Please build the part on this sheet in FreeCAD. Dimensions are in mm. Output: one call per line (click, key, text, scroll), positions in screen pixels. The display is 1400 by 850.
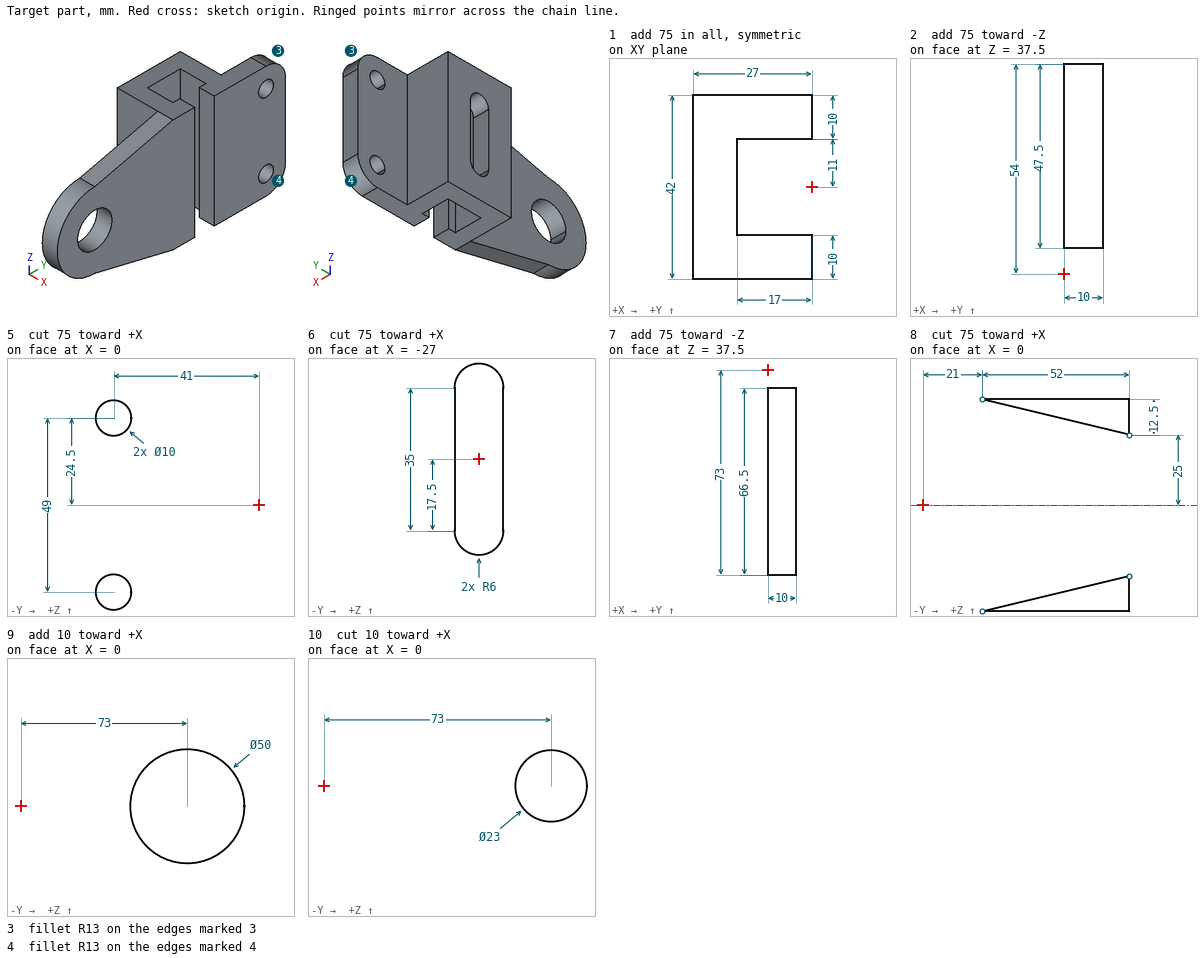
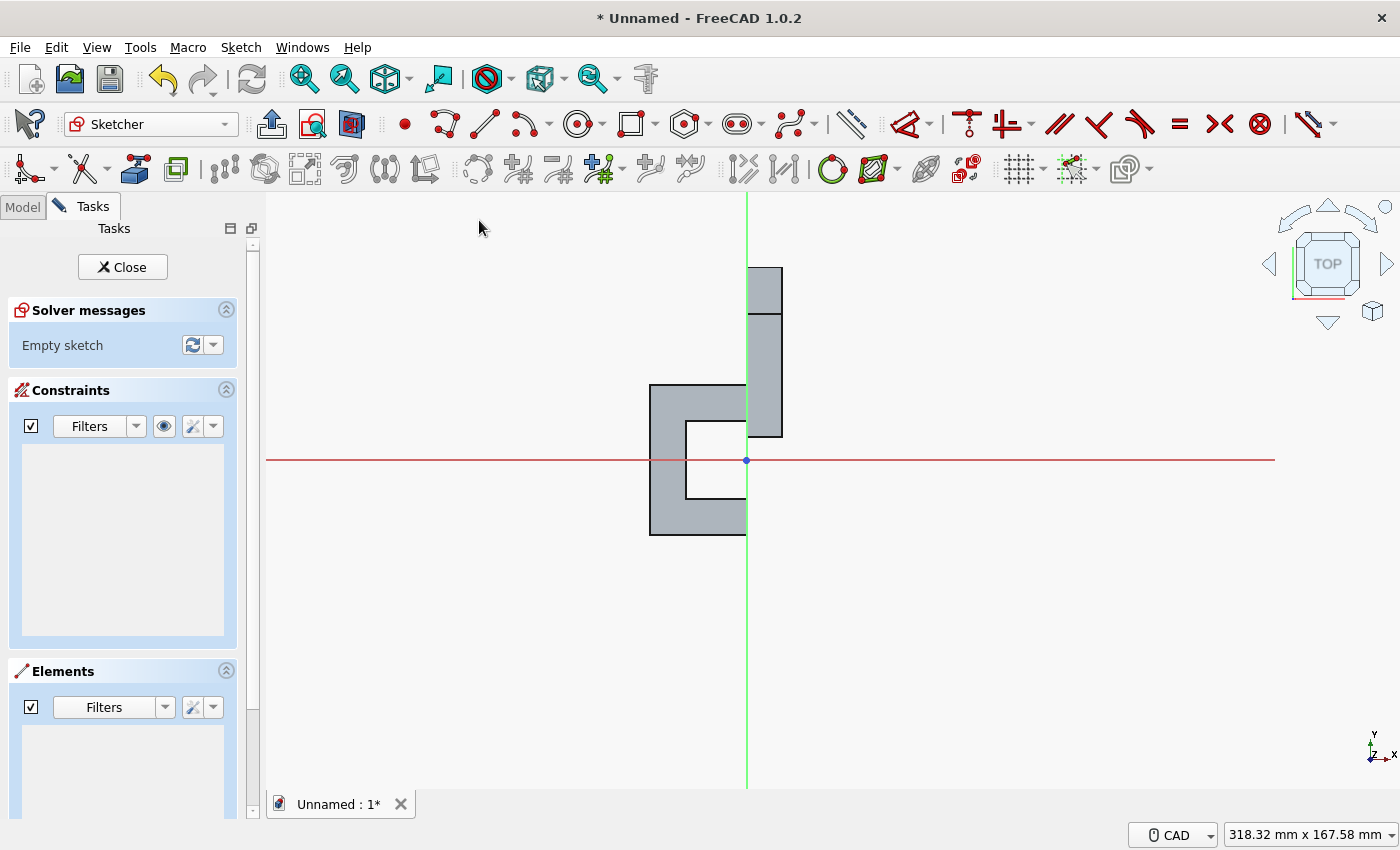
scroll(764, 761, up, 2)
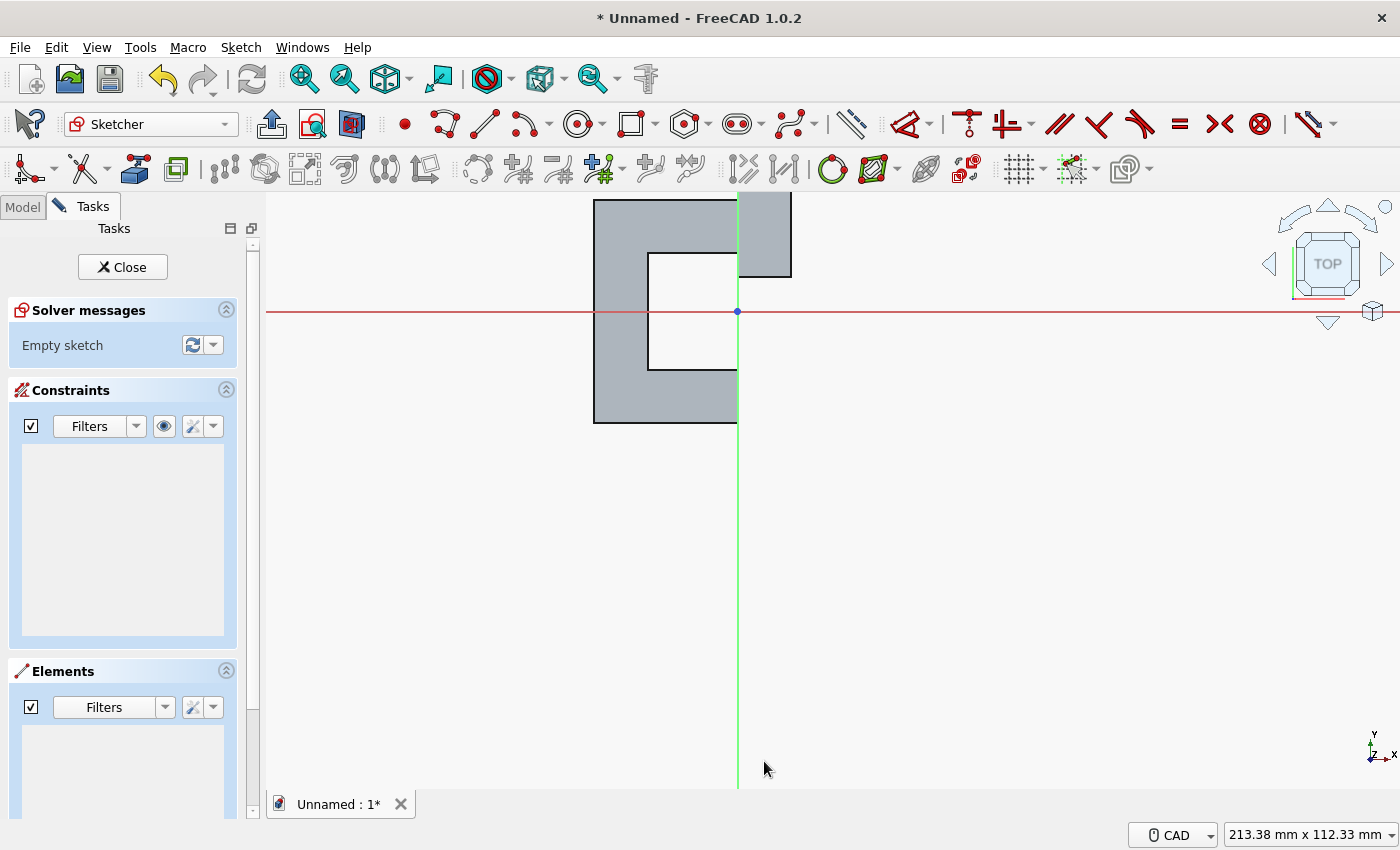
key(g)
key(r)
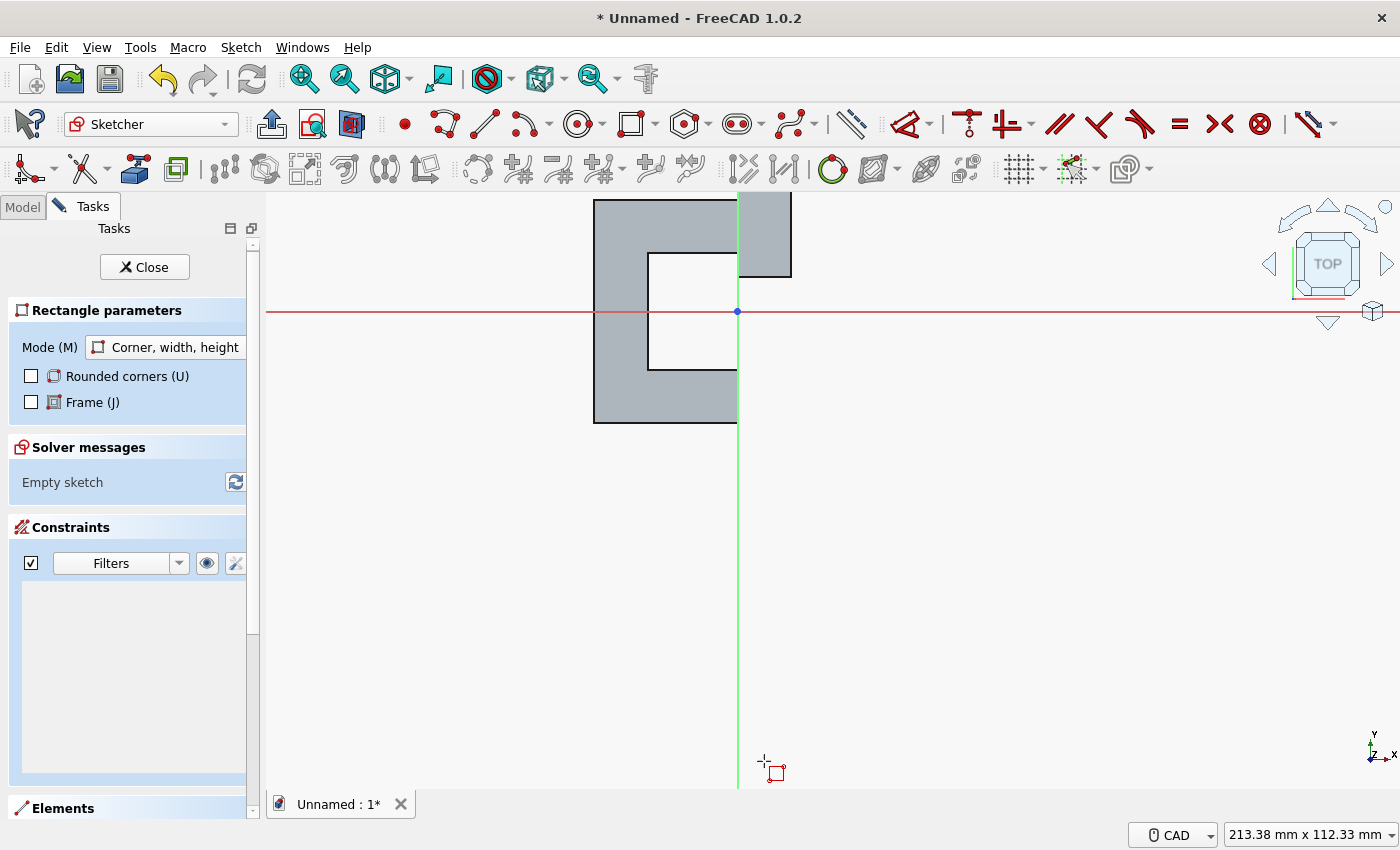
click(738, 346)
click(791, 700)
key(Escape)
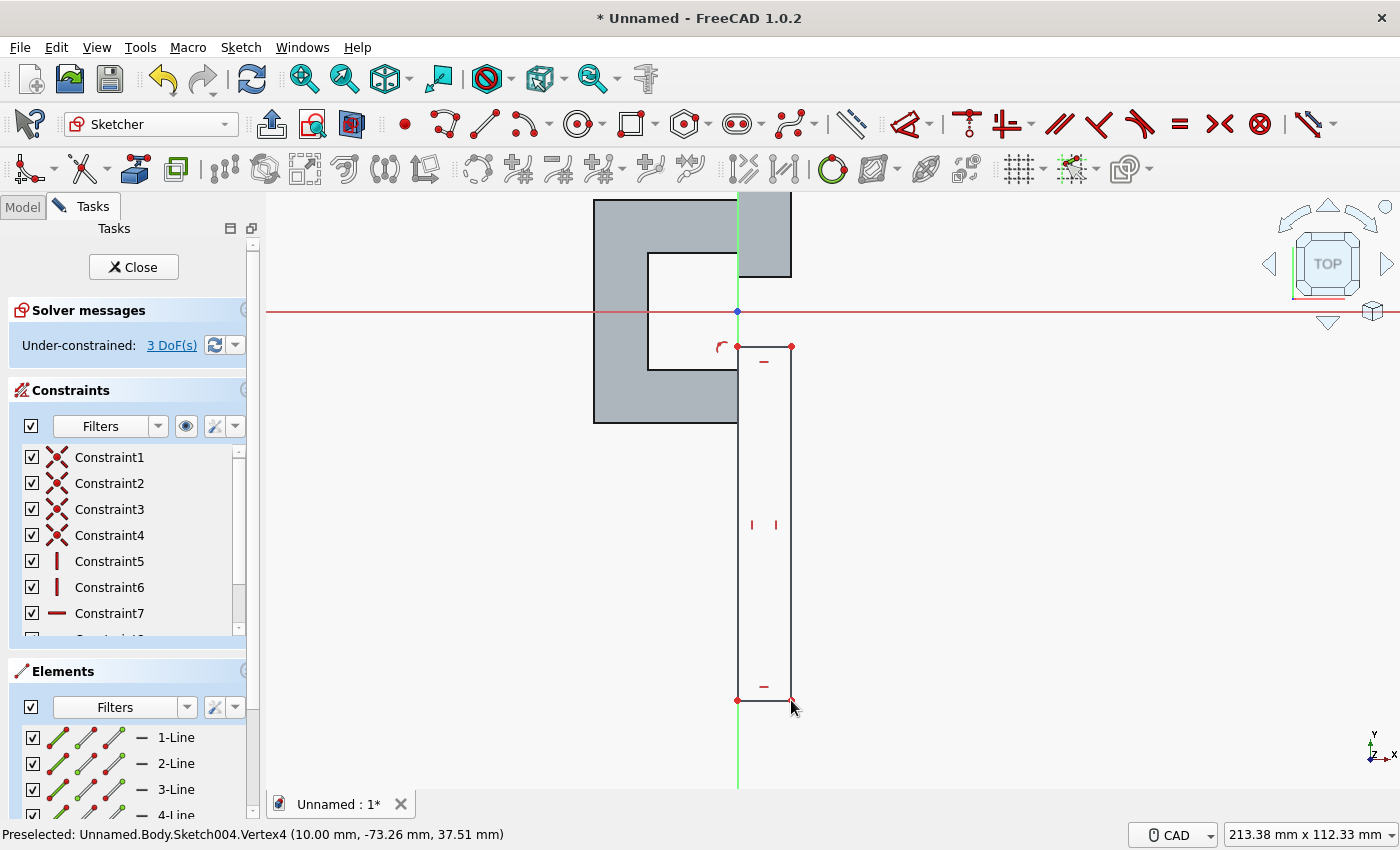
key(d)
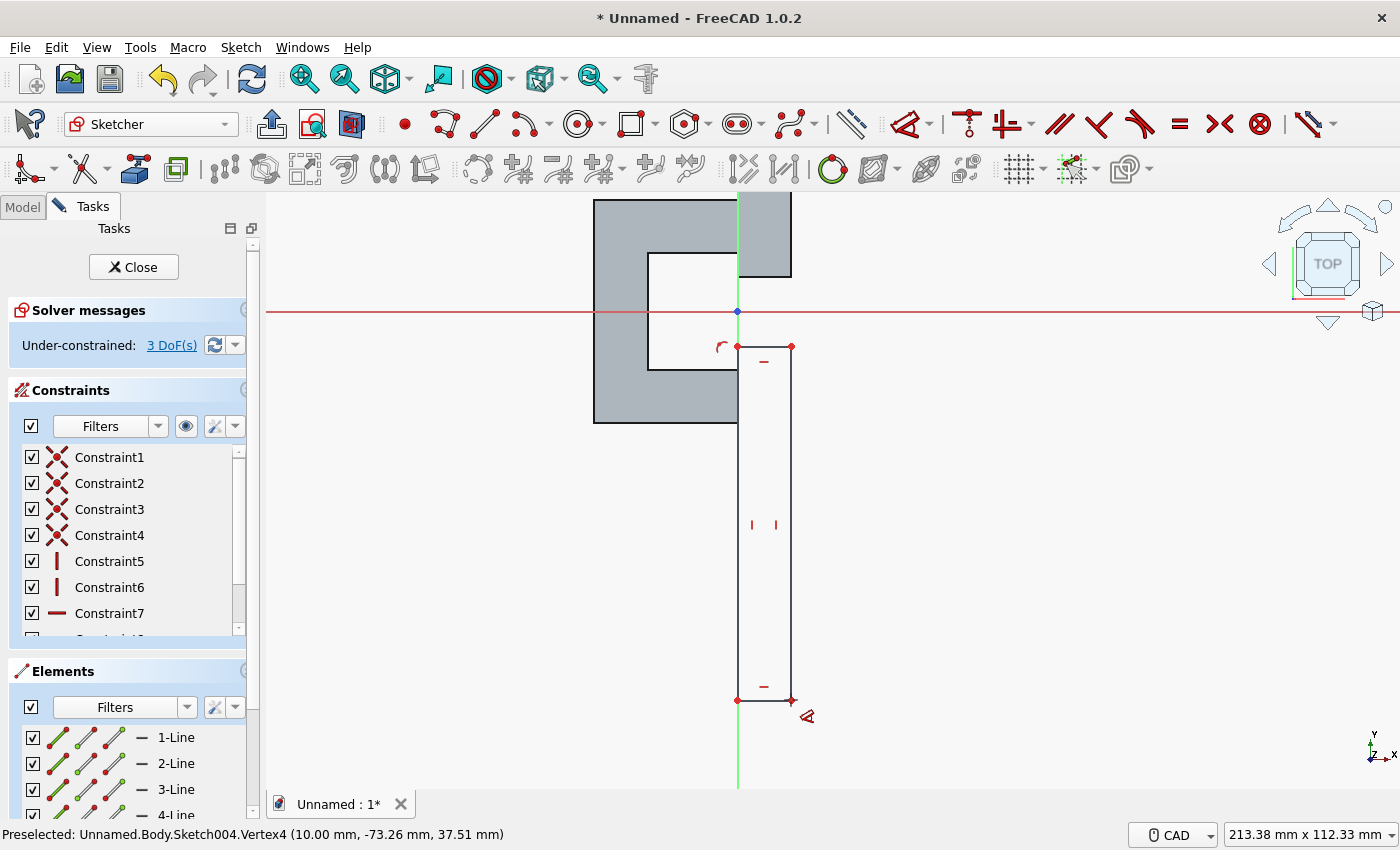
click(754, 701)
click(764, 735)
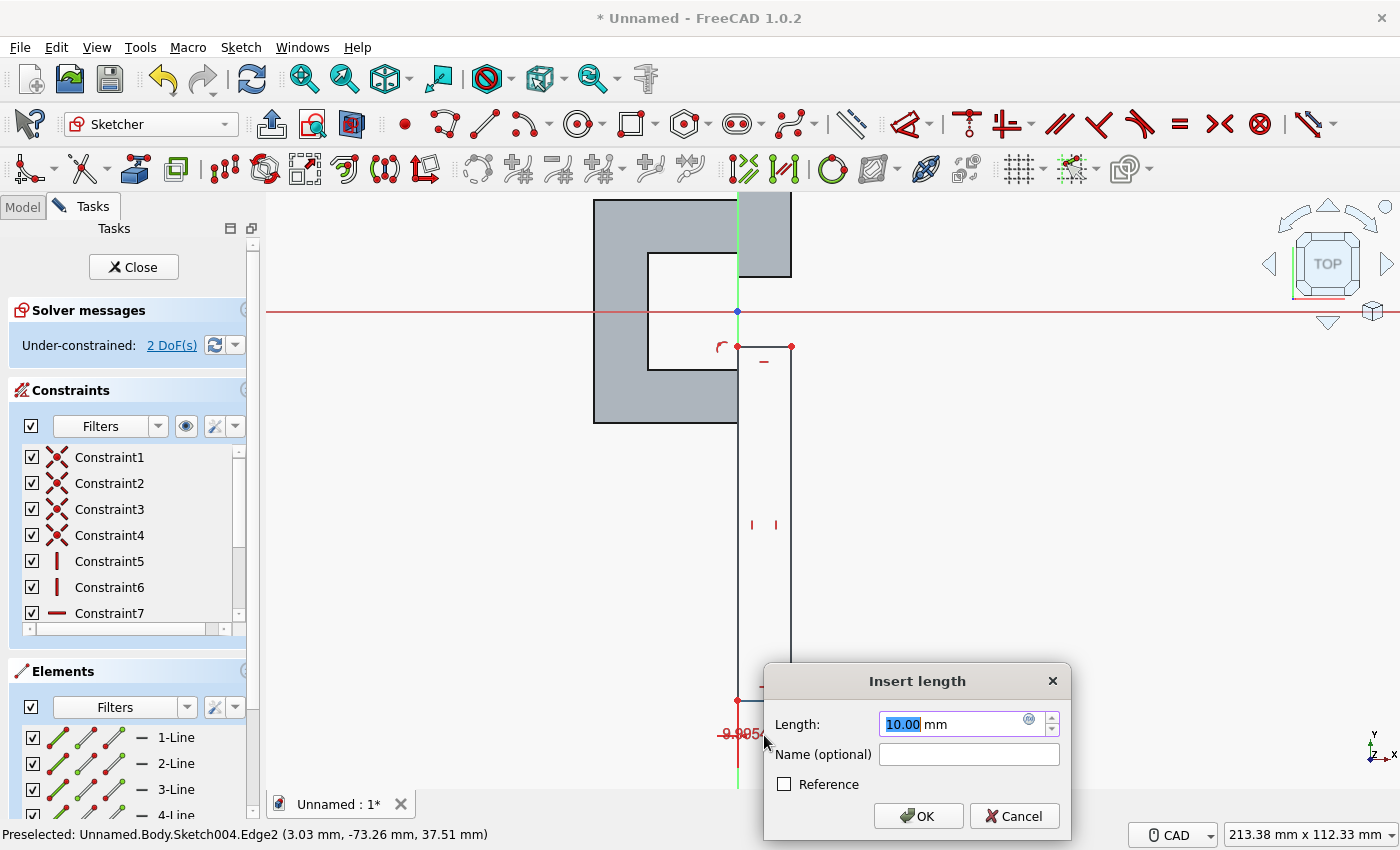
text(10)
key(Return)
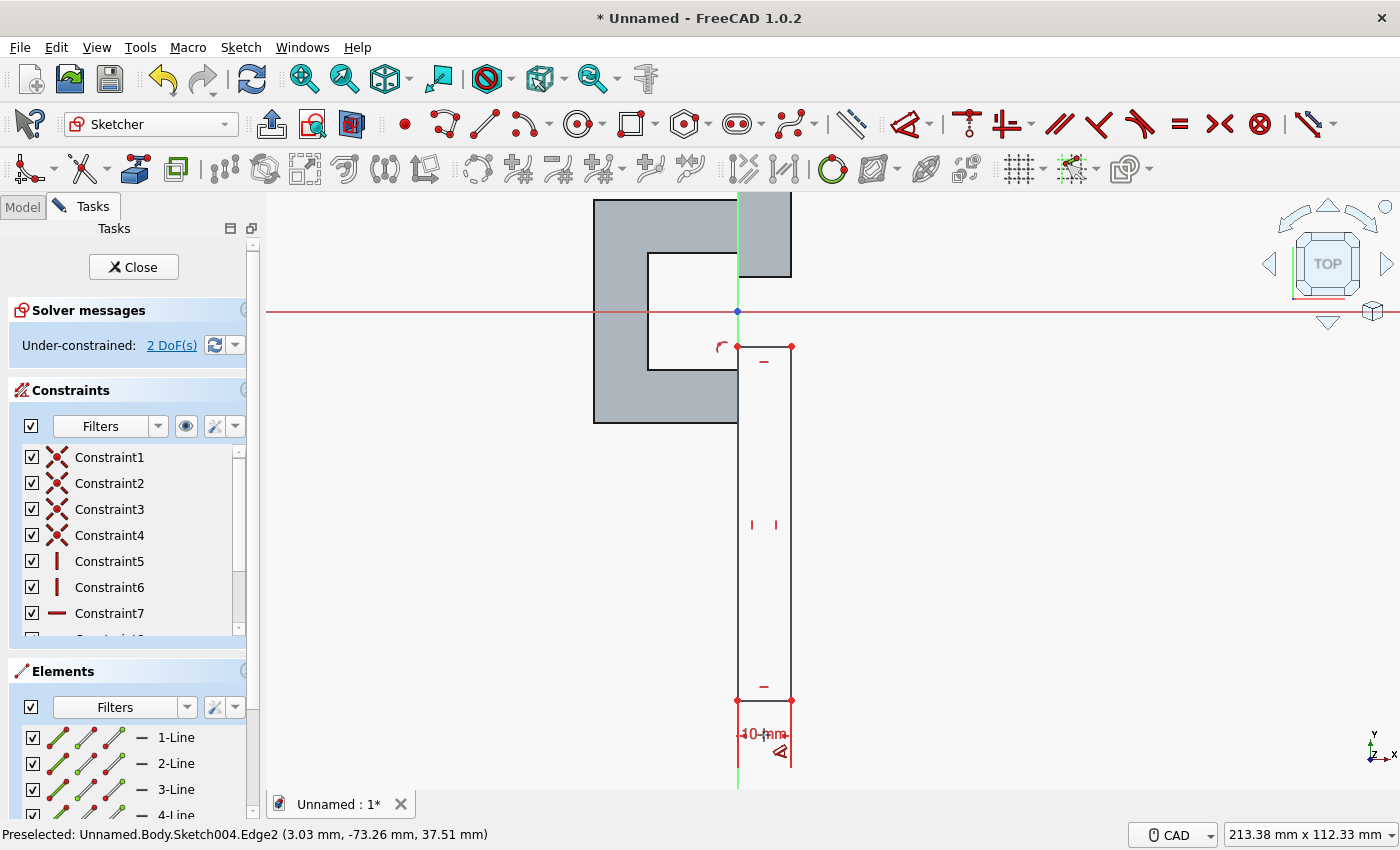
click(738, 701)
click(704, 506)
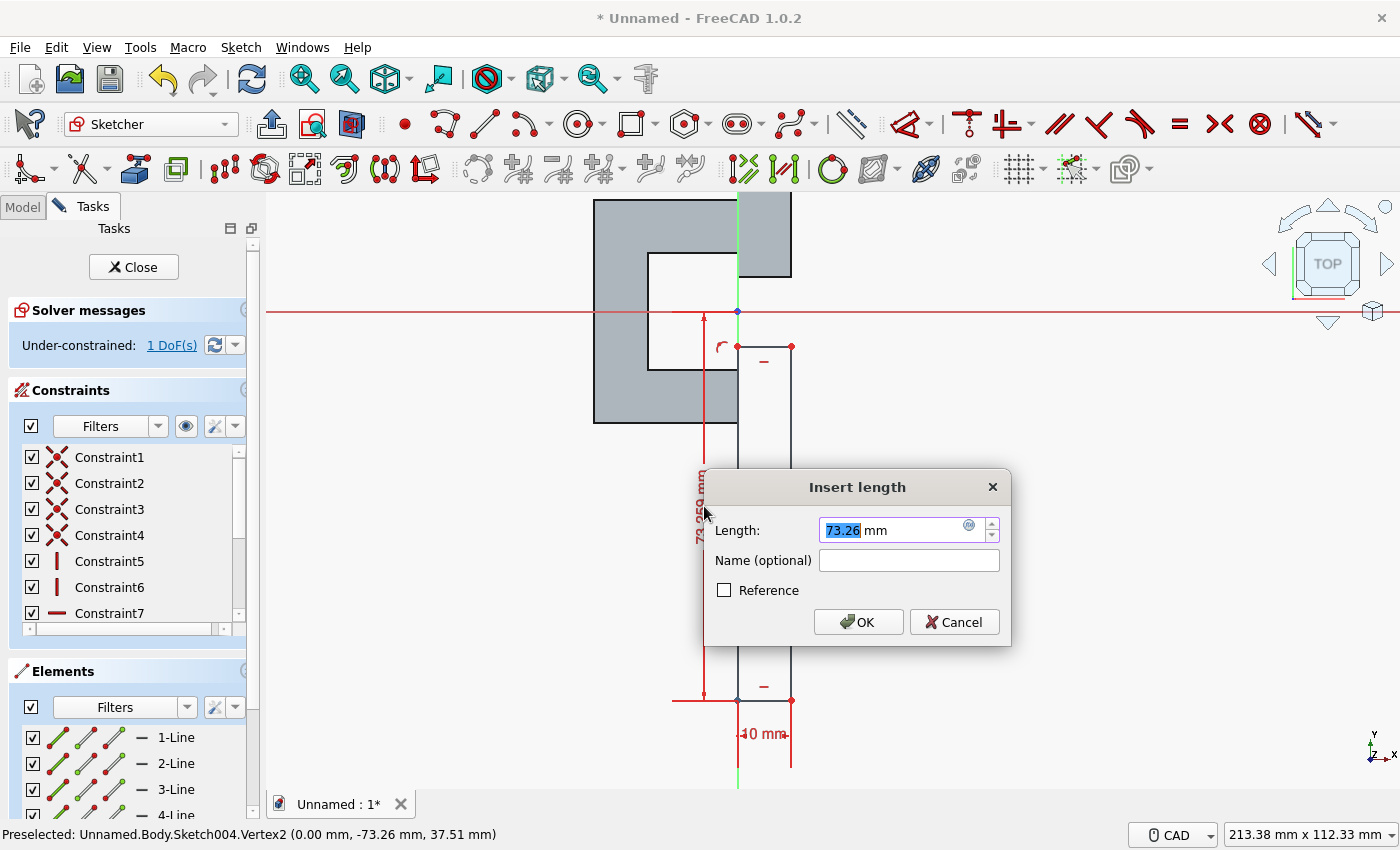
text(73)
key(Return)